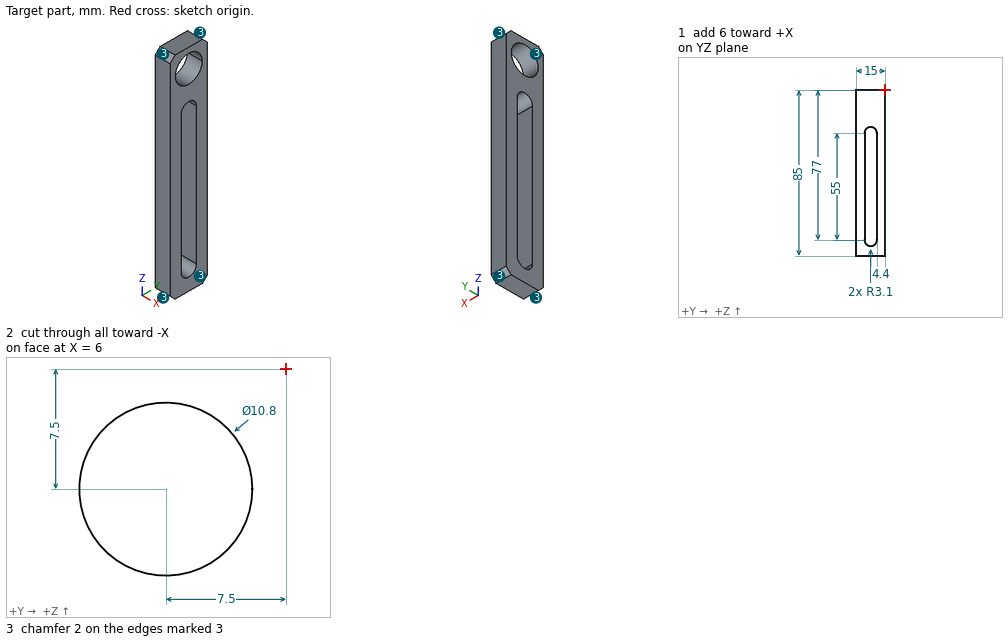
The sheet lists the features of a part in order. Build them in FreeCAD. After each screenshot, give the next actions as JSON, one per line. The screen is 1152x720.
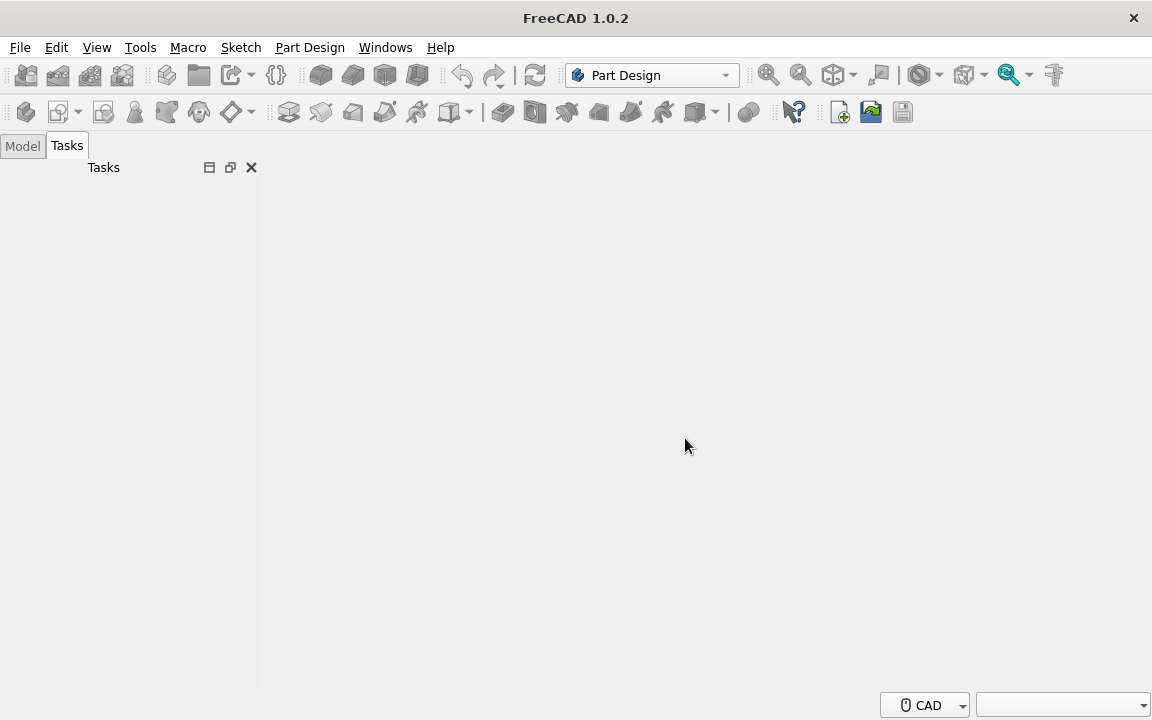
{"action": "left_click", "coordinate": [840, 112]}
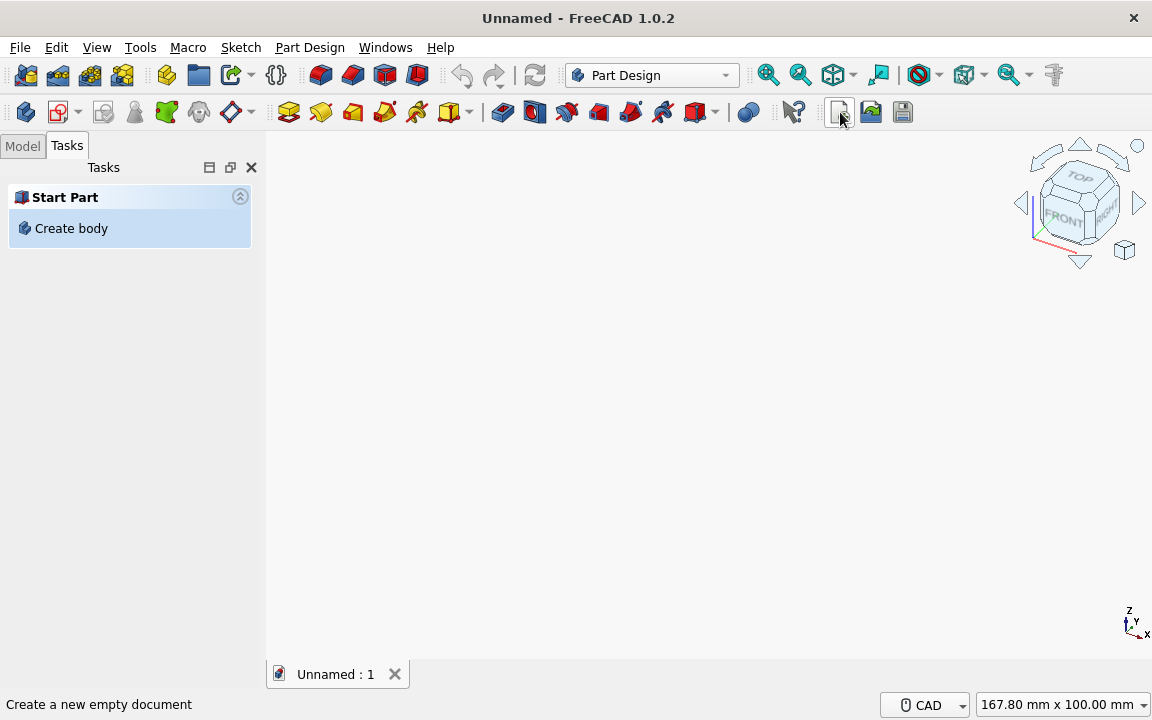
{"action": "left_click", "coordinate": [58, 112]}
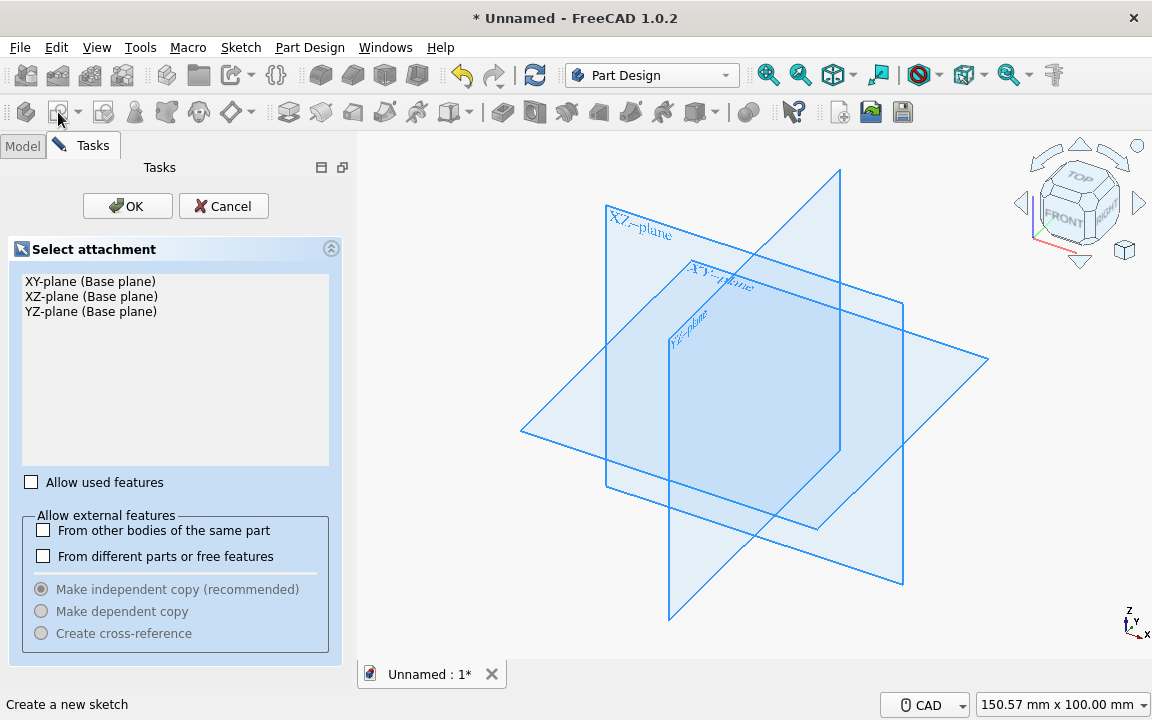
{"action": "left_click", "coordinate": [82, 312]}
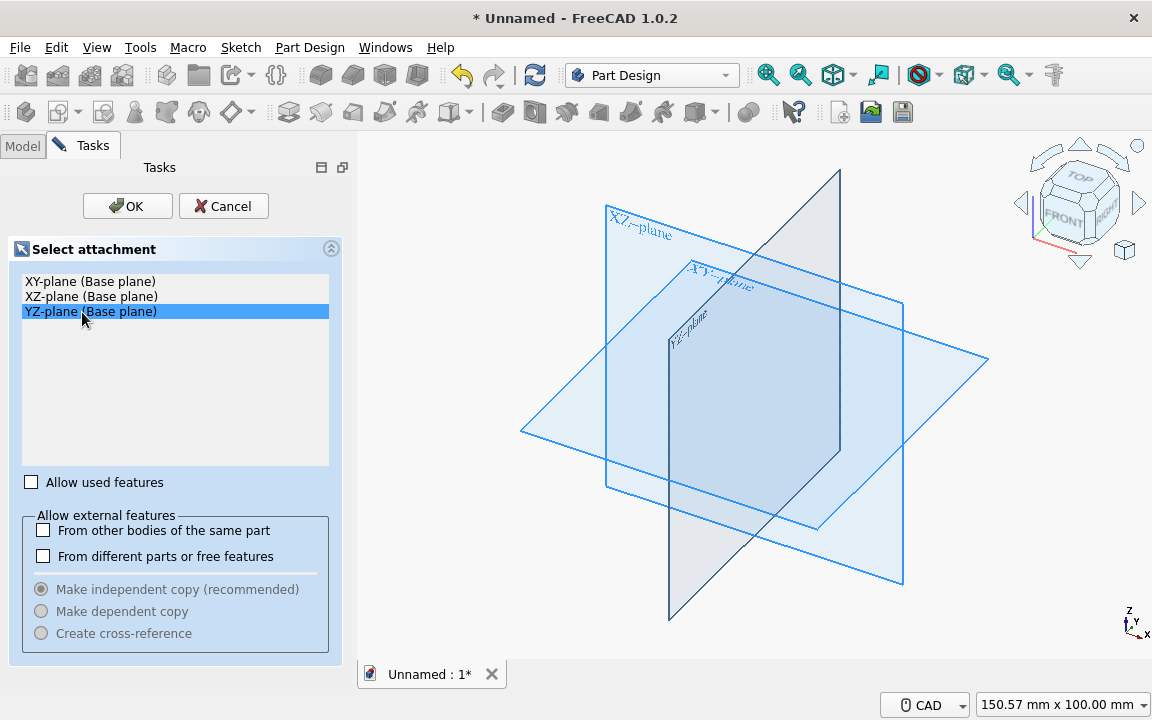
{"action": "left_click", "coordinate": [128, 206]}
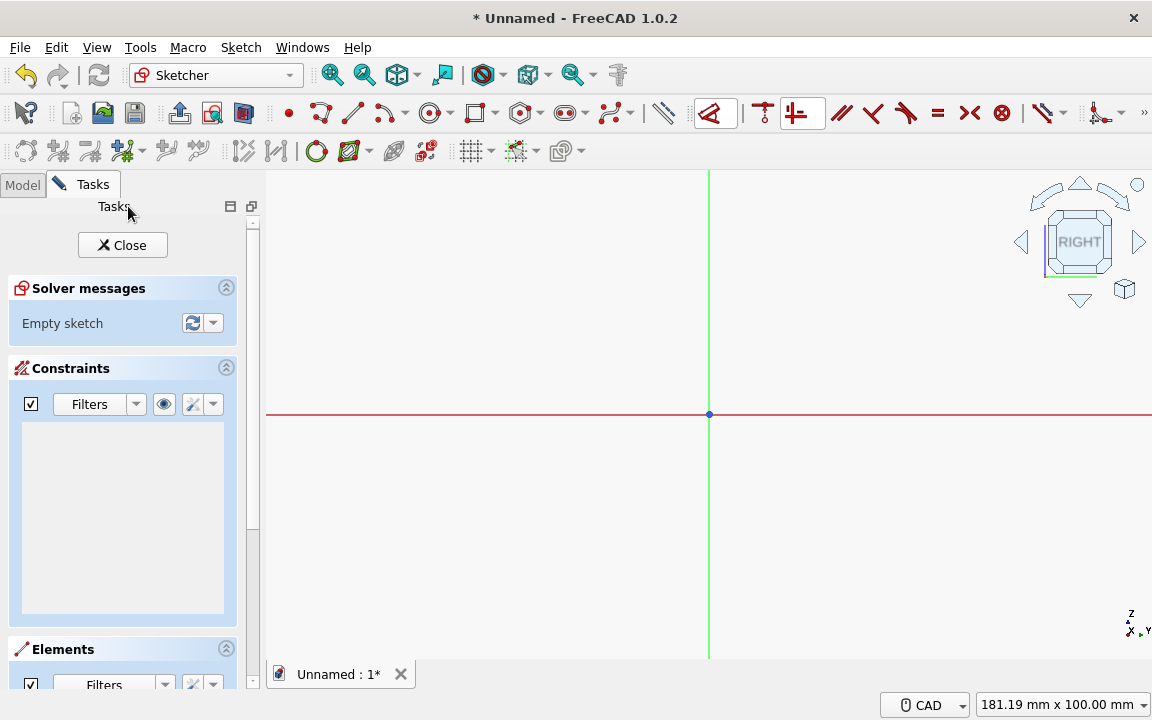
{"action": "scroll", "coordinate": [602, 198], "scroll_direction": "down", "scroll_amount": 3}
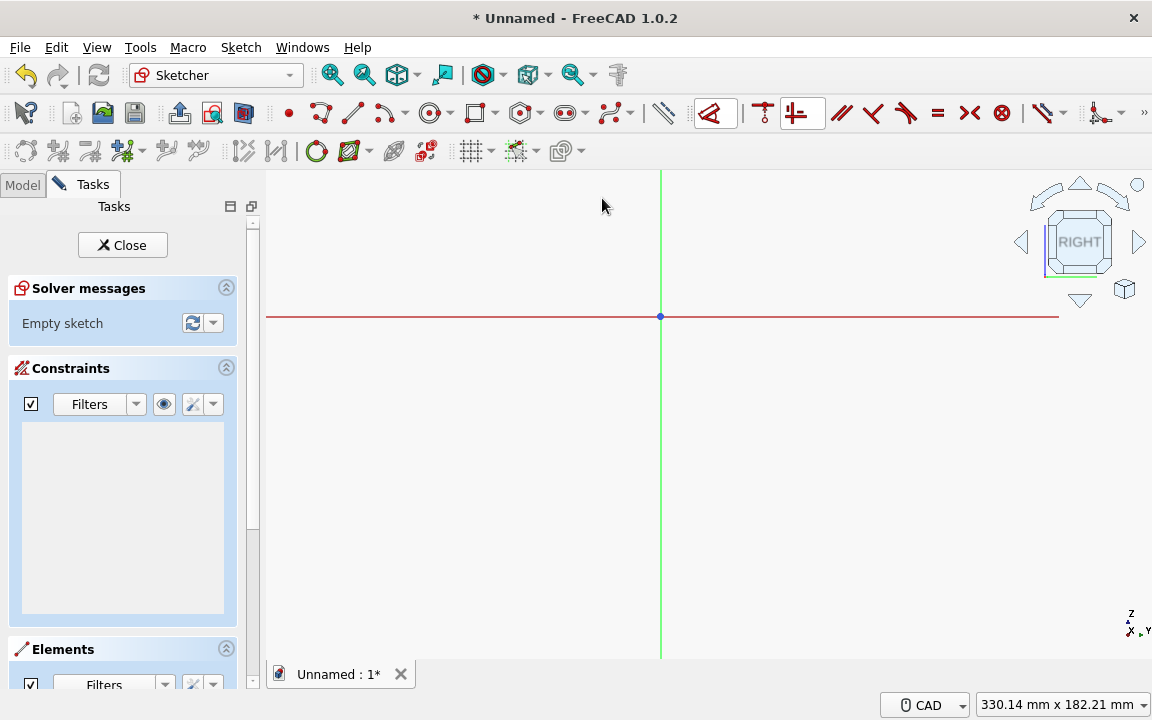
{"action": "left_click", "coordinate": [476, 114]}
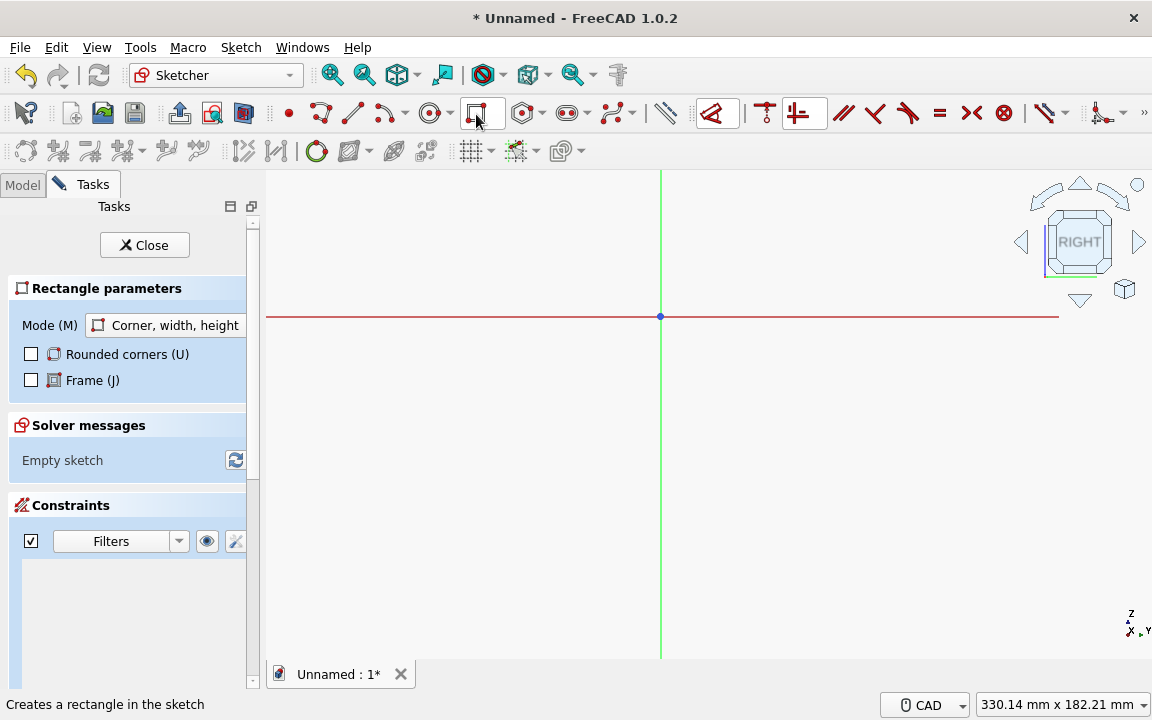
{"action": "left_click", "coordinate": [661, 317]}
{"action": "left_click", "coordinate": [621, 545]}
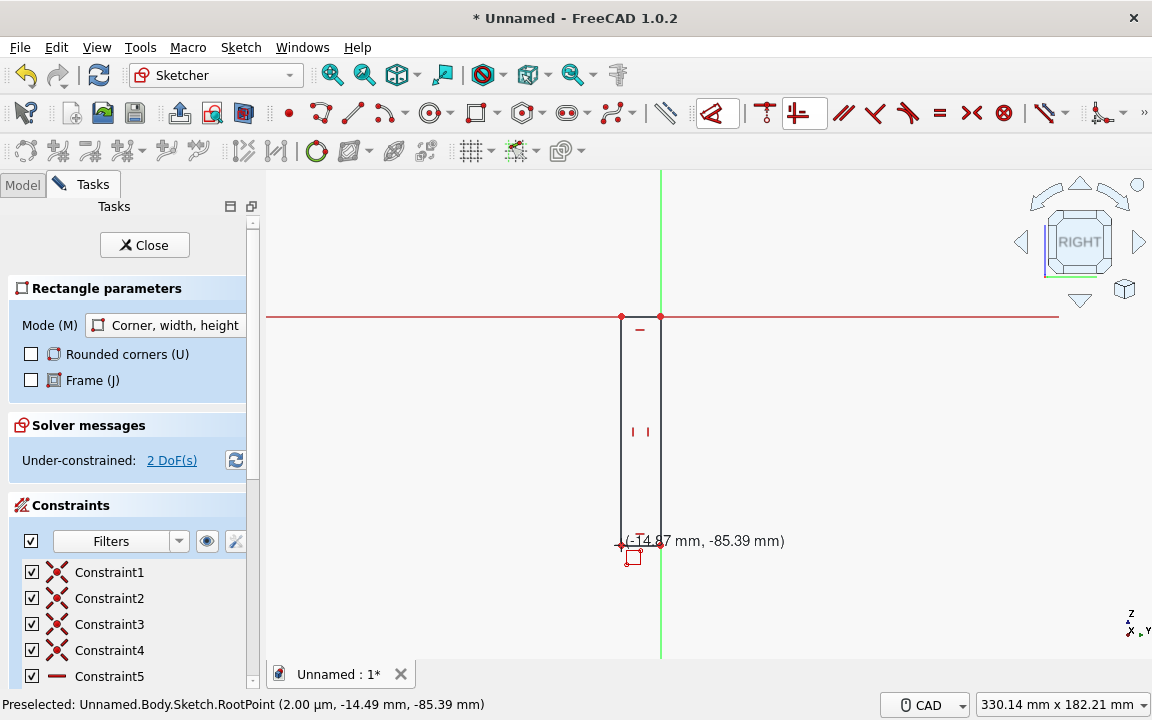
{"action": "left_click", "coordinate": [568, 114]}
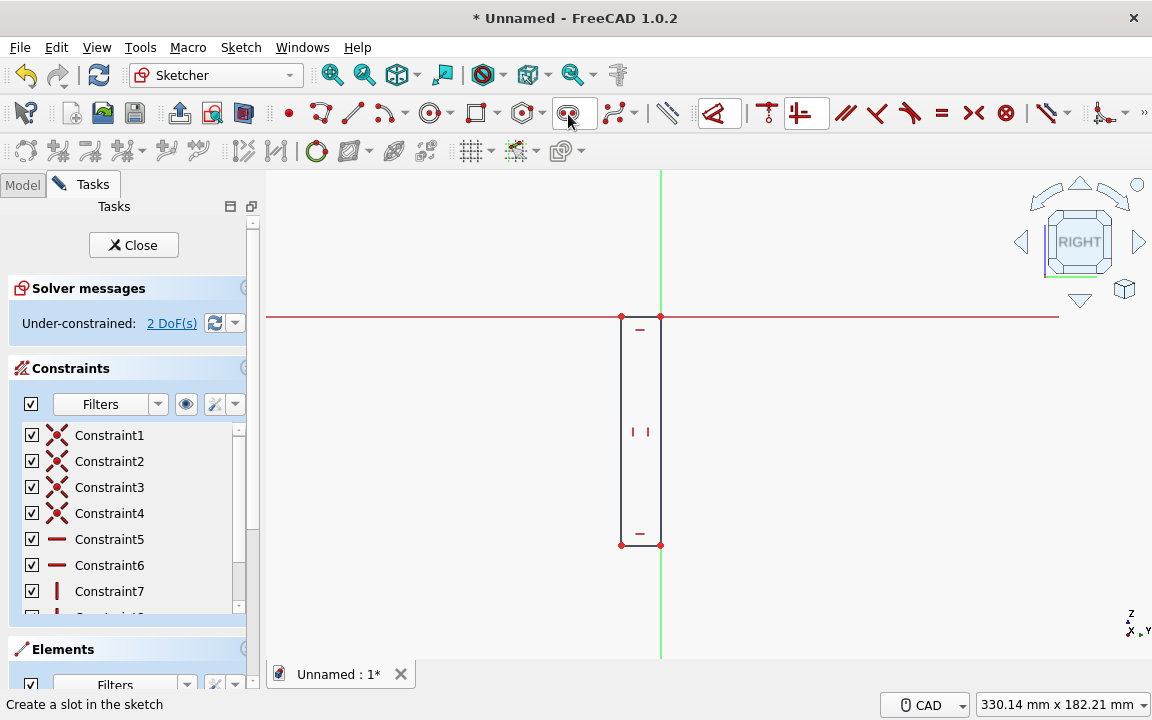
{"action": "scroll", "coordinate": [641, 523], "scroll_direction": "up", "scroll_amount": 6}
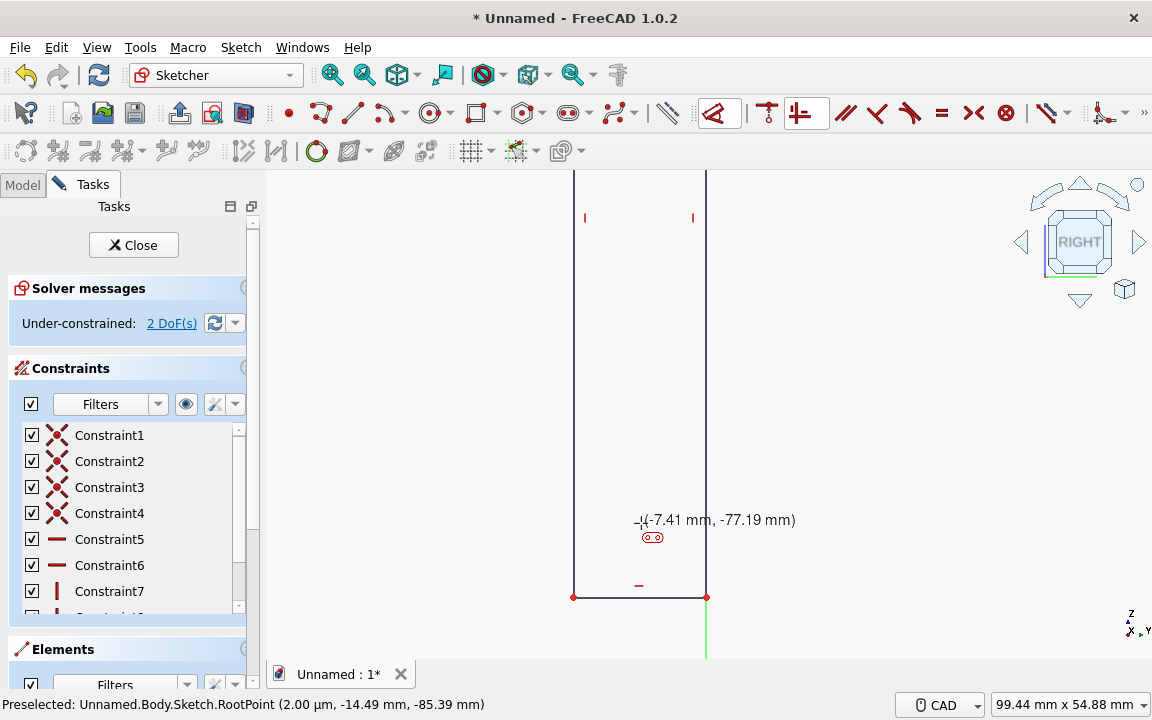
{"action": "left_click", "coordinate": [639, 523]}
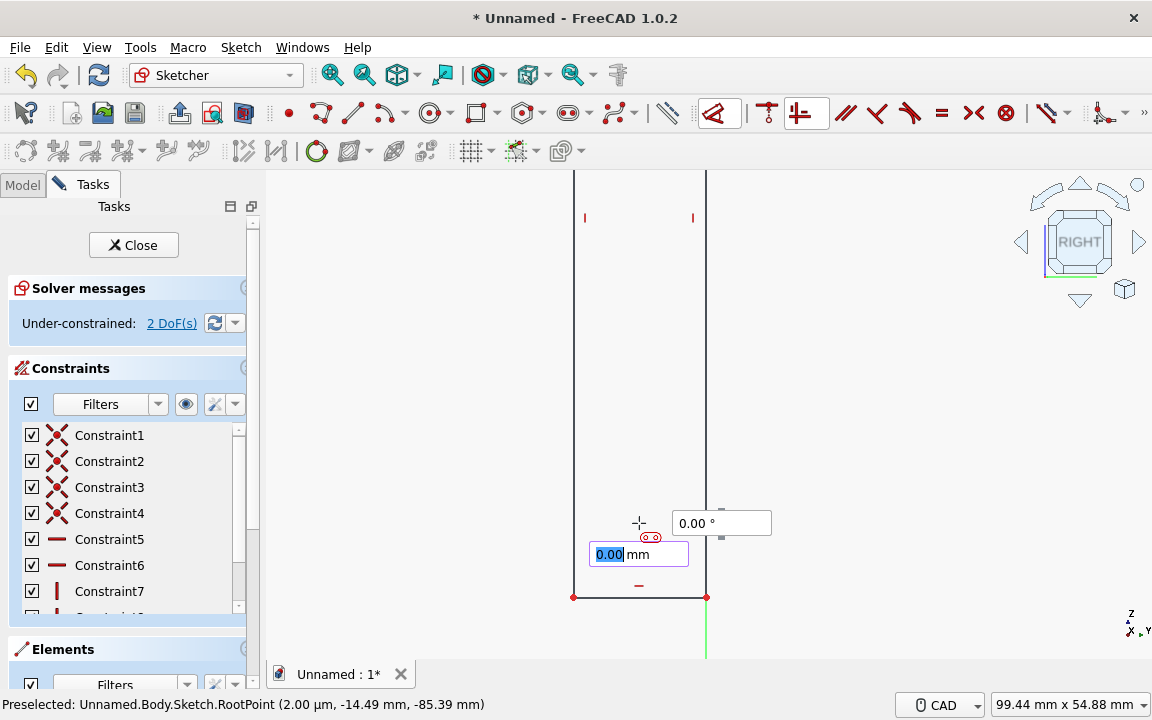
{"action": "scroll", "coordinate": [641, 530], "scroll_direction": "down", "scroll_amount": 5}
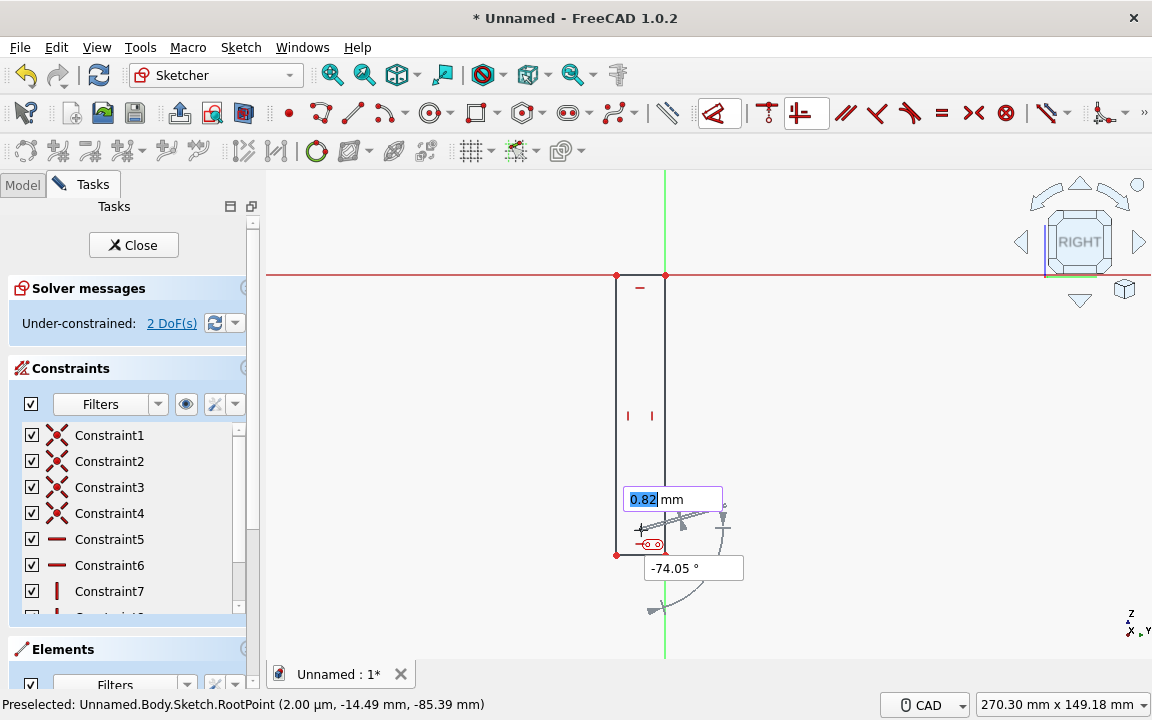
{"action": "left_click", "coordinate": [641, 348]}